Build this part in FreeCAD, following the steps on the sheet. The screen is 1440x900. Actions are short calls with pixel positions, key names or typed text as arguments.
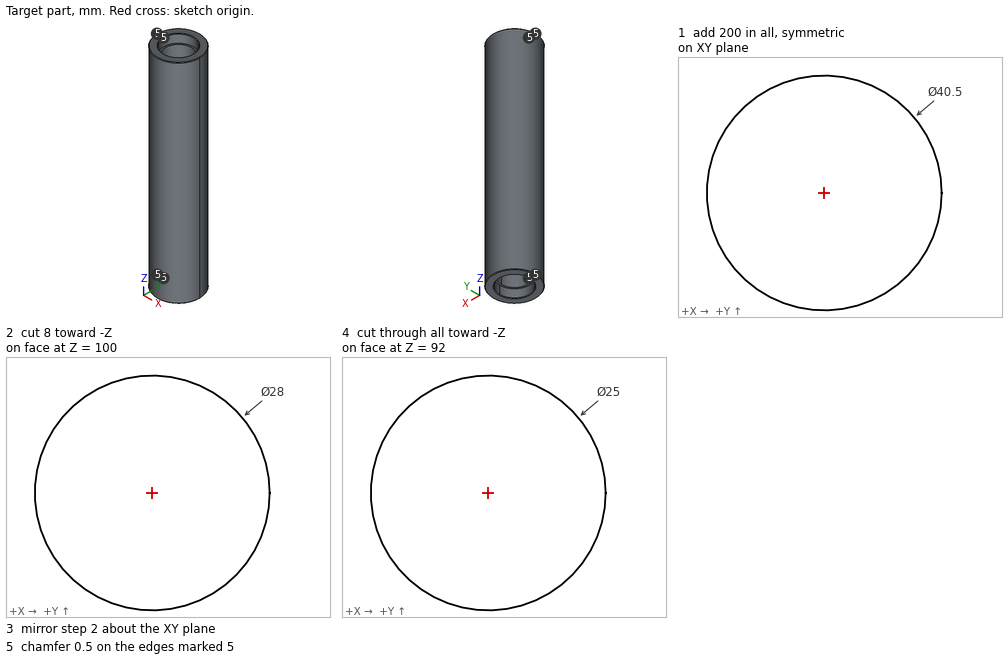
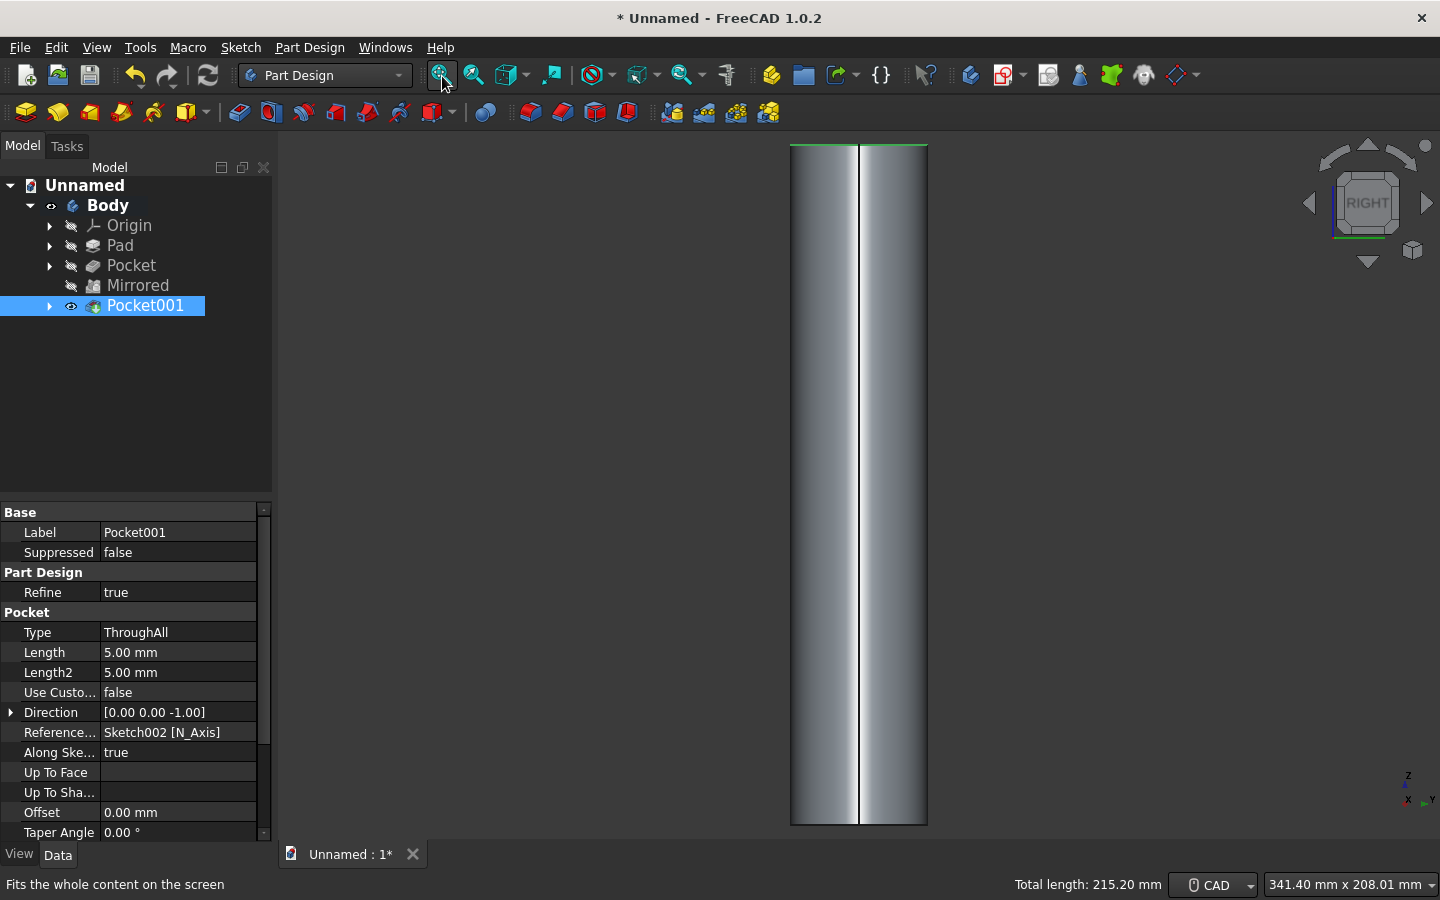
key(5)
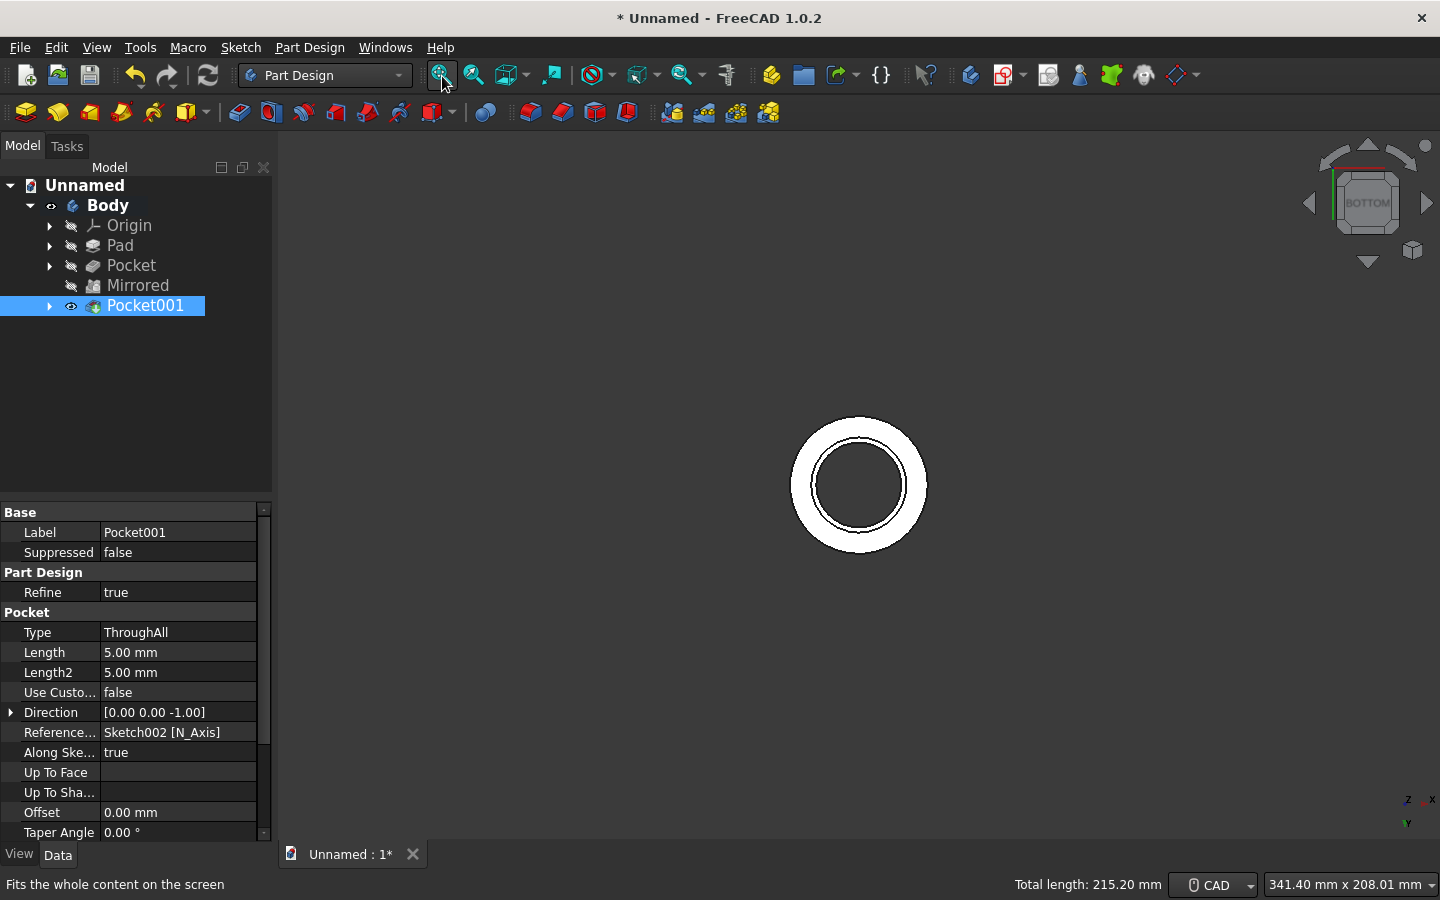
click(442, 76)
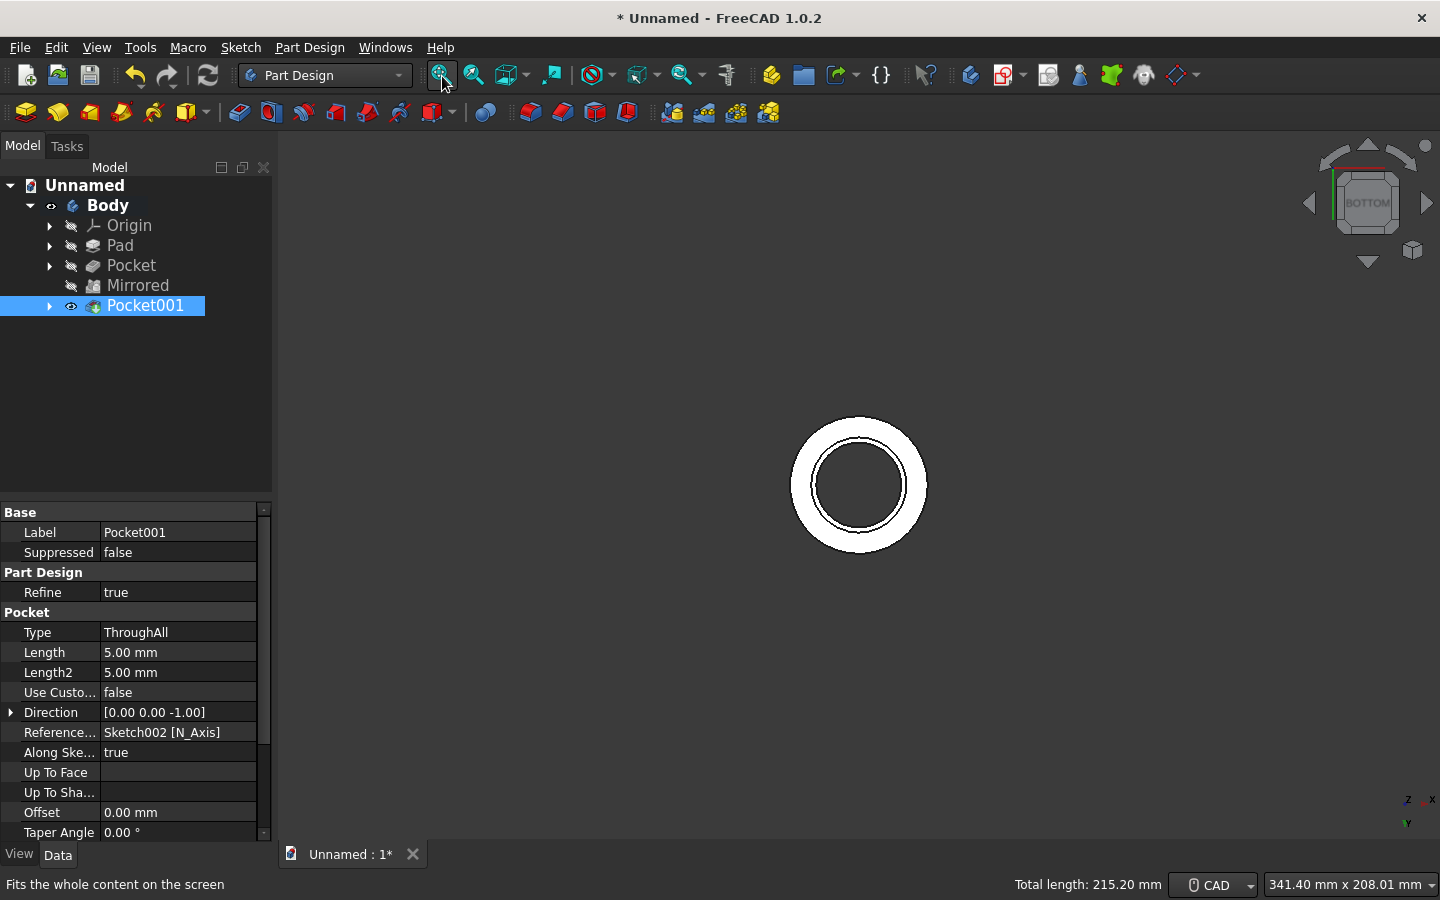
click(811, 484, ctrl)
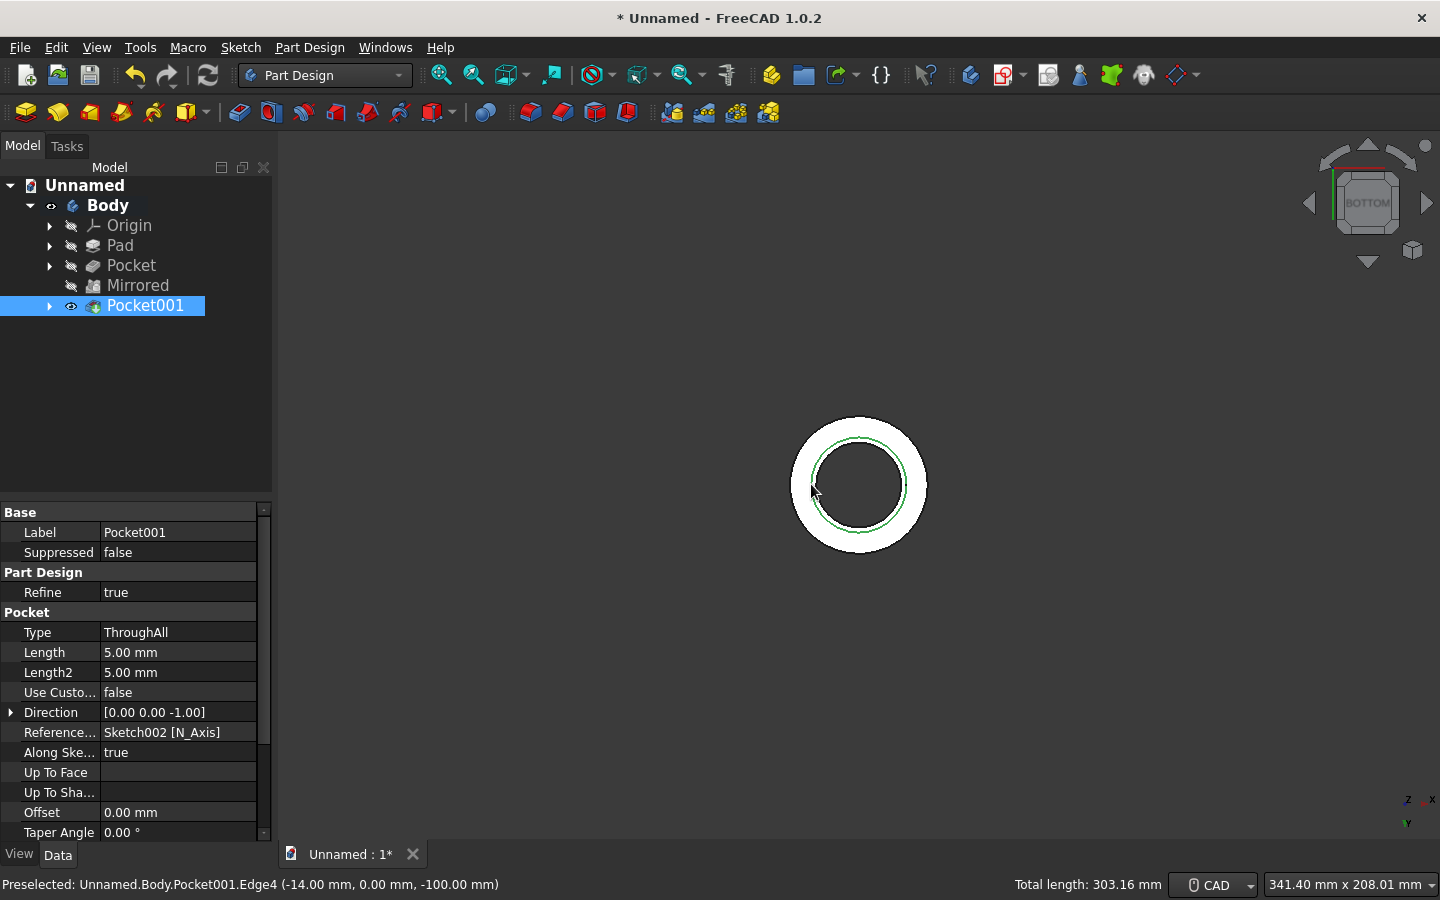
click(790, 484, ctrl)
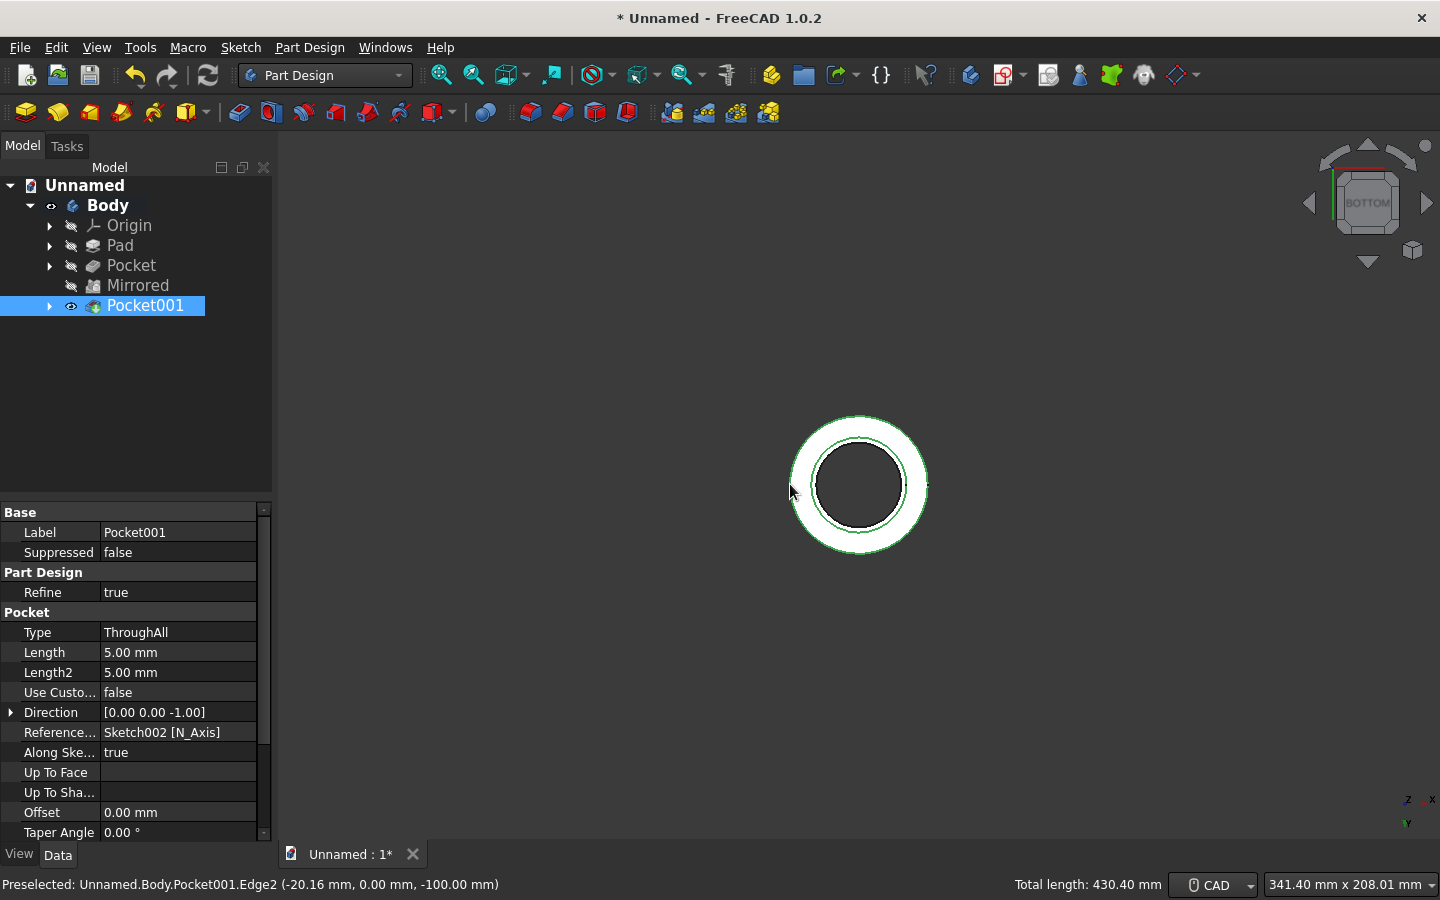
click(564, 112)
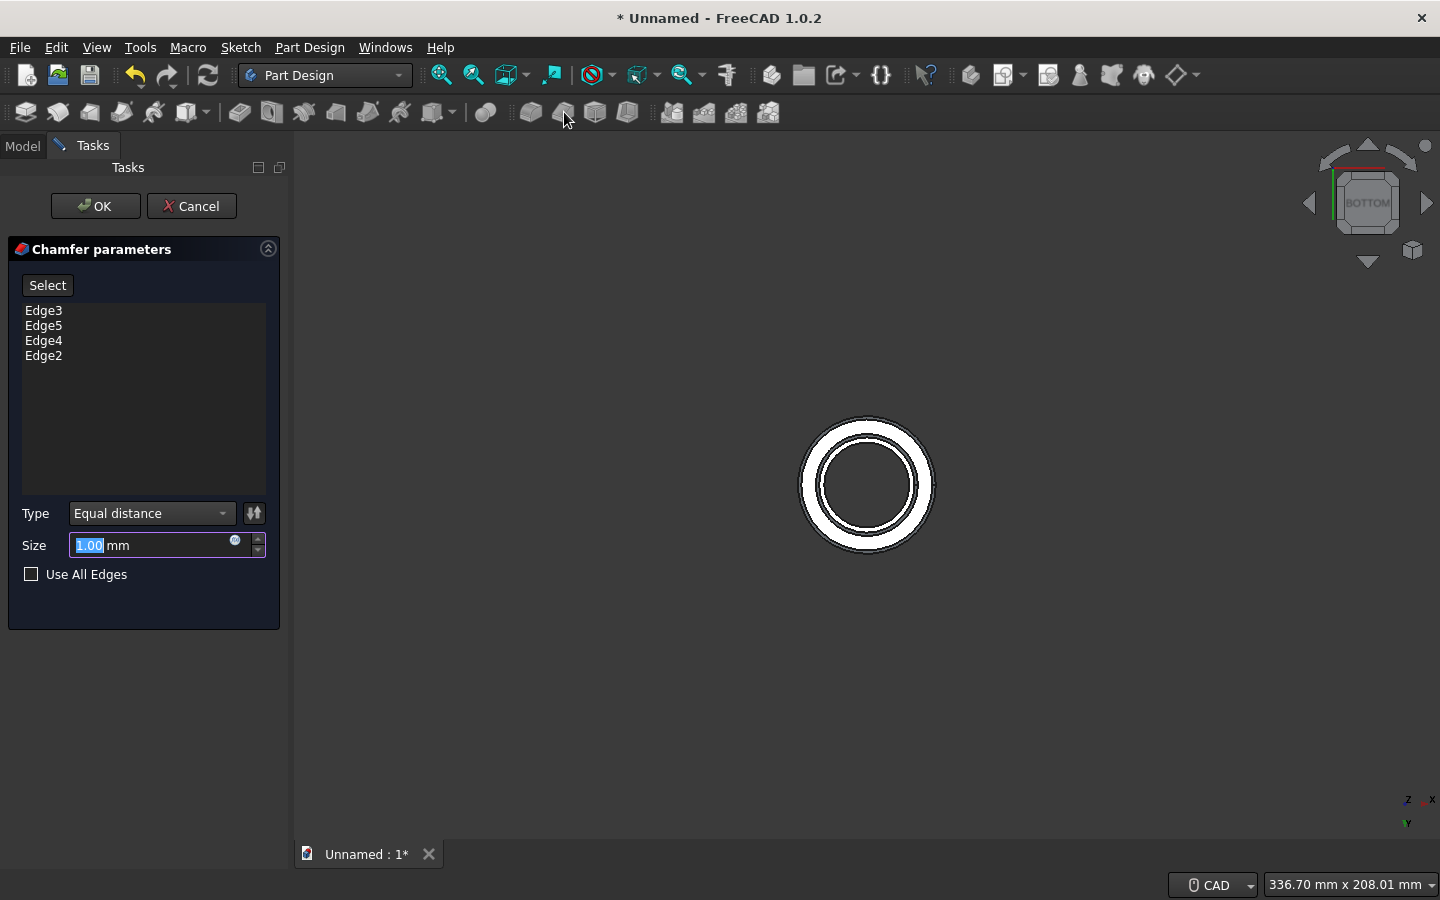
text(0.5)
key(Tab)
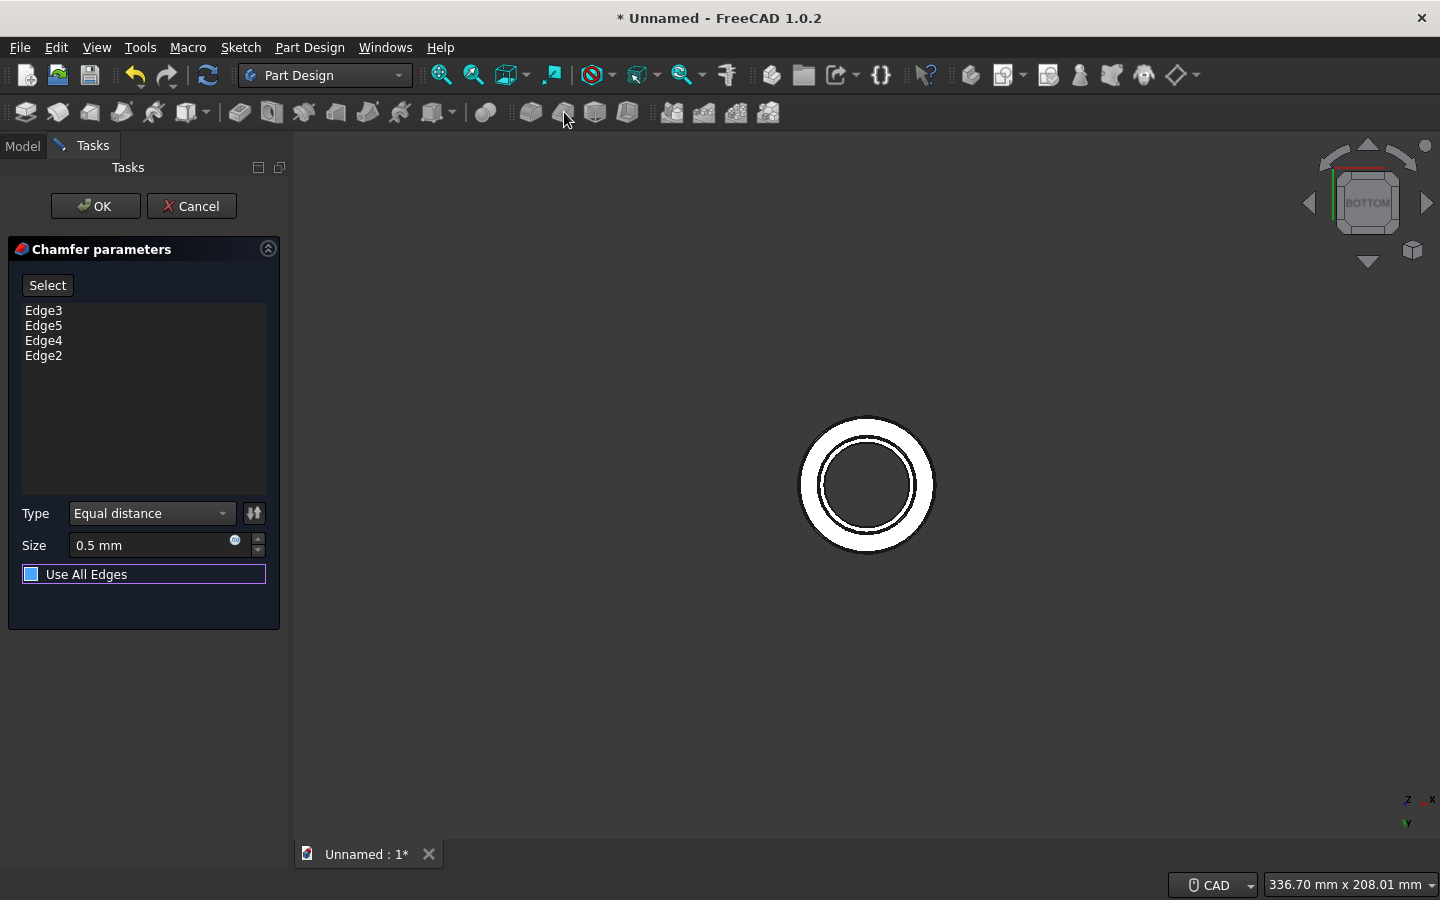
click(96, 206)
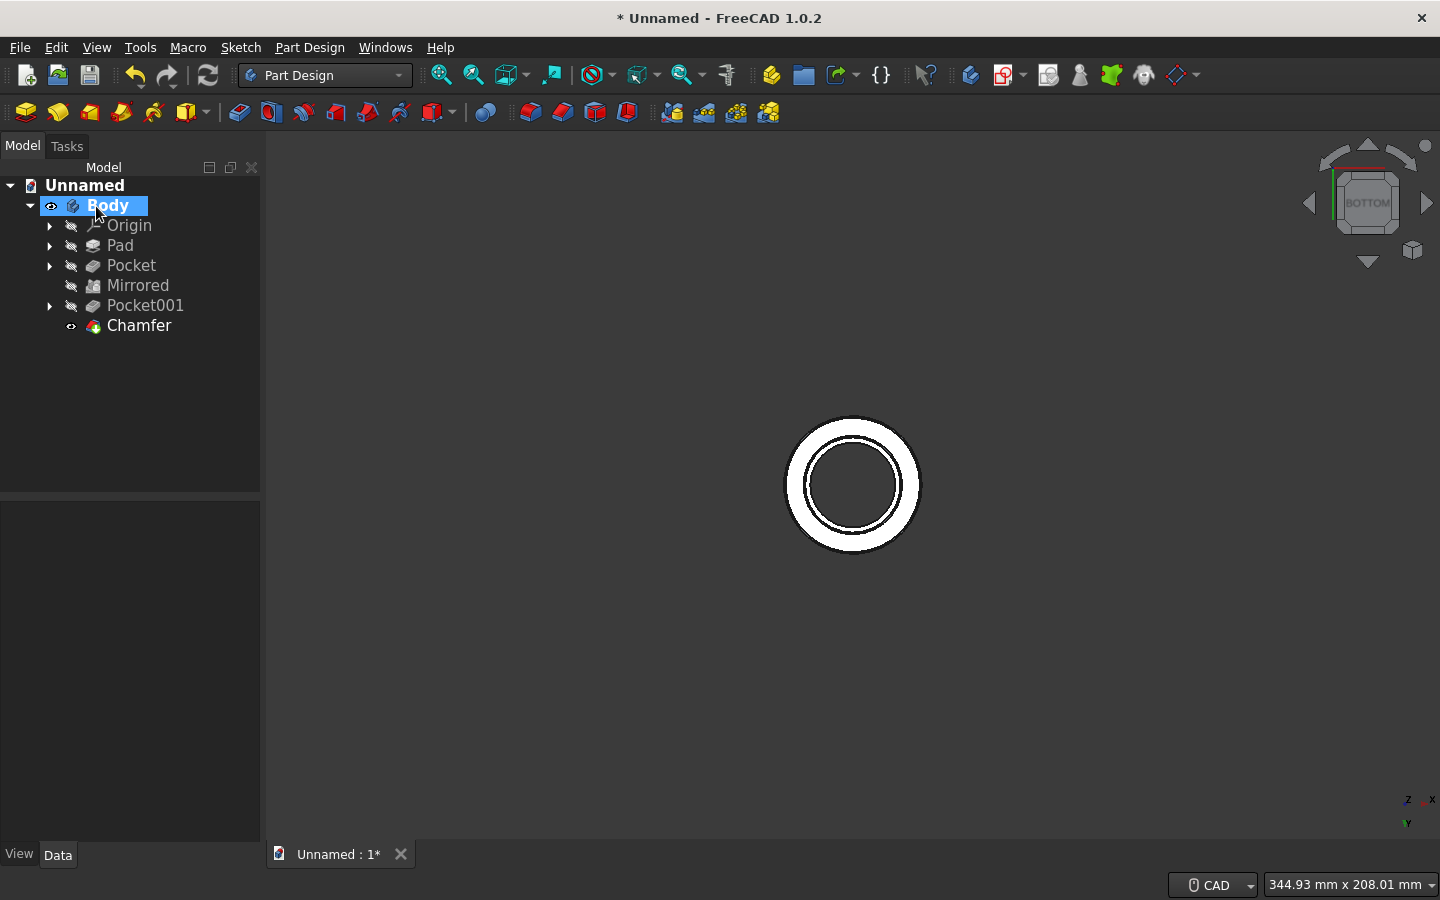
key(0)